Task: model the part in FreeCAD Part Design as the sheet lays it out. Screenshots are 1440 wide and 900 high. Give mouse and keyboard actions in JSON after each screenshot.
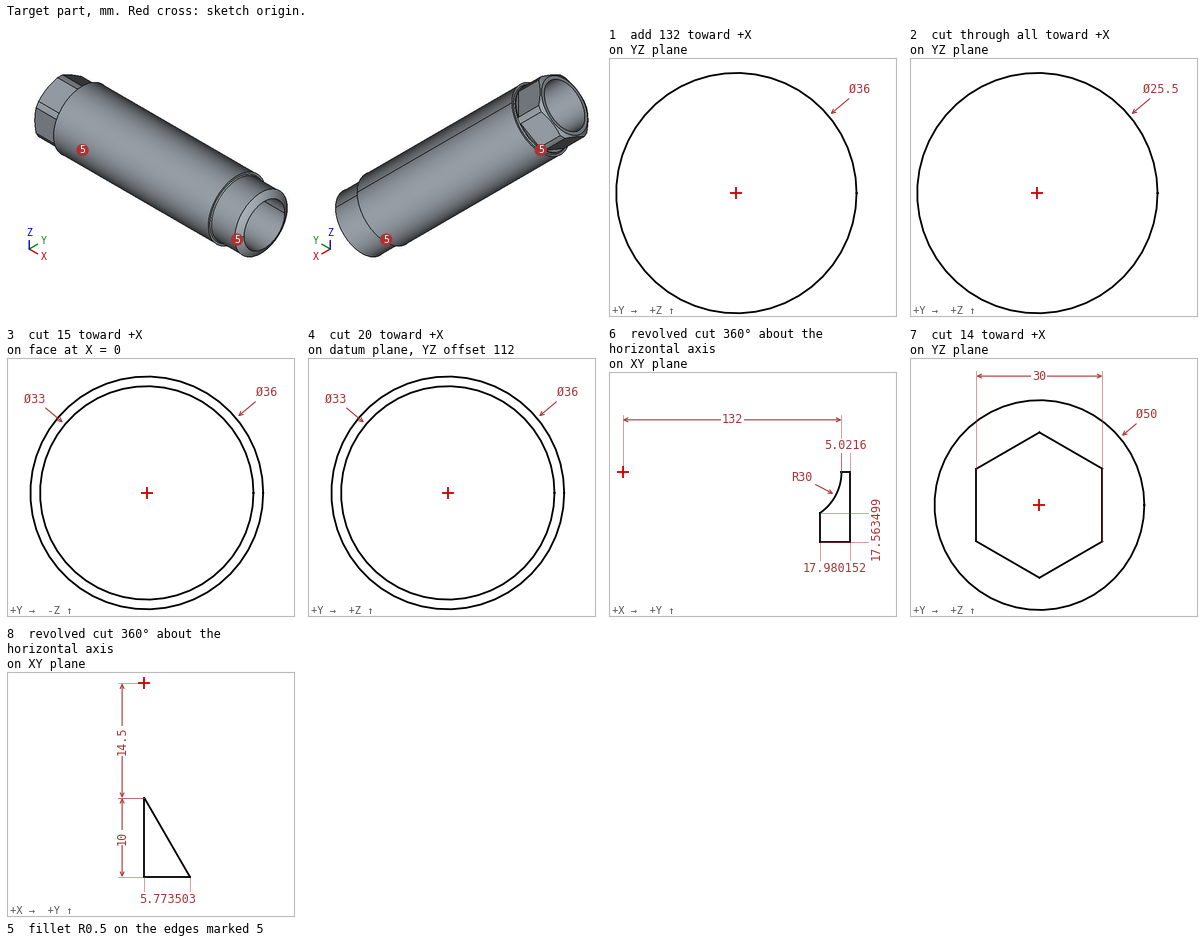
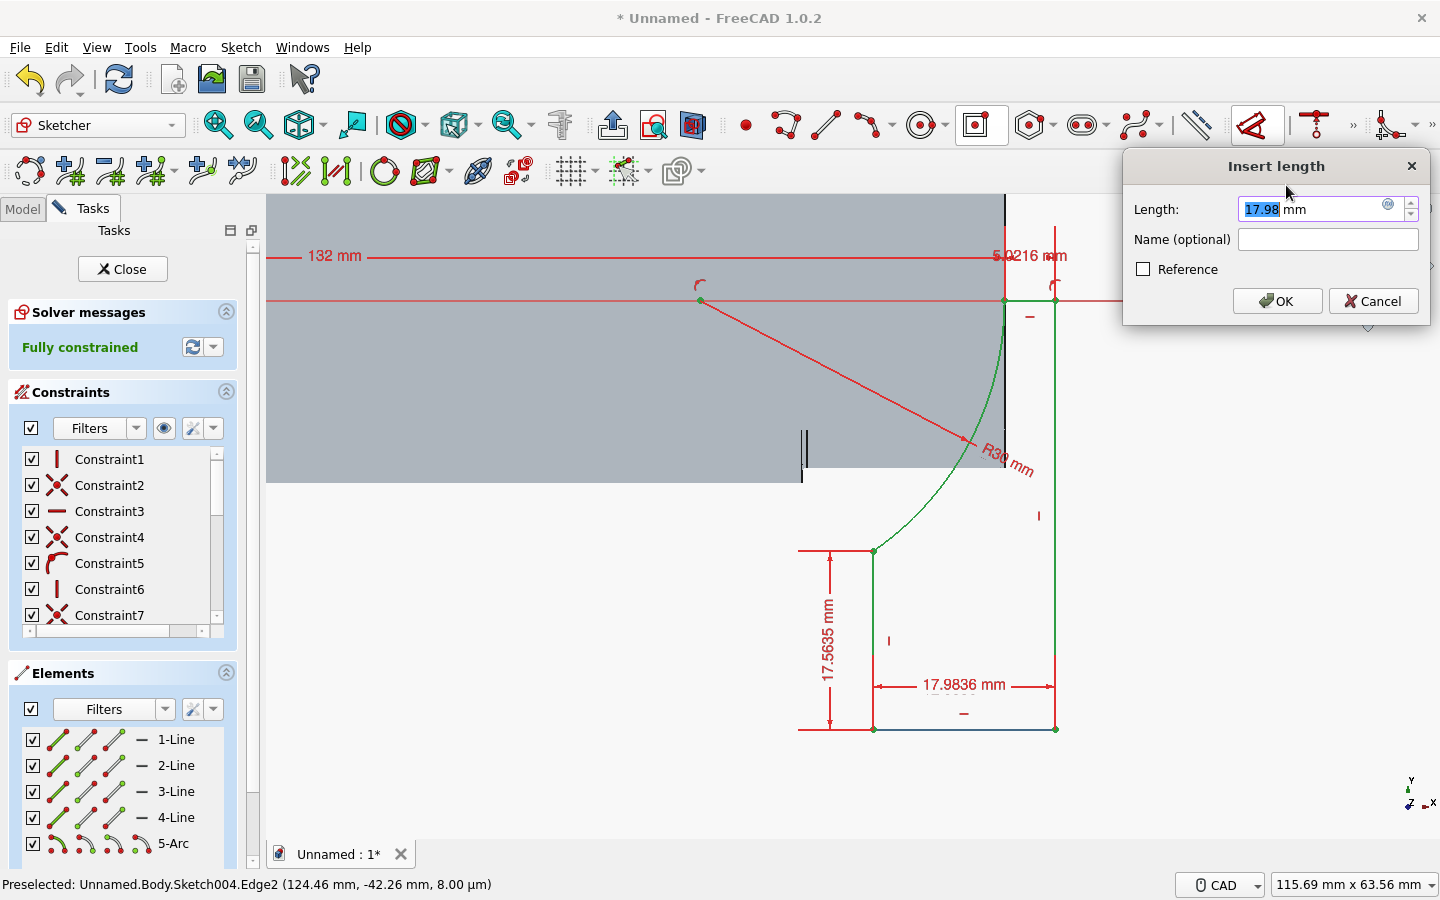
{"action": "type", "text": "17.980152"}
{"action": "key", "text": "Return"}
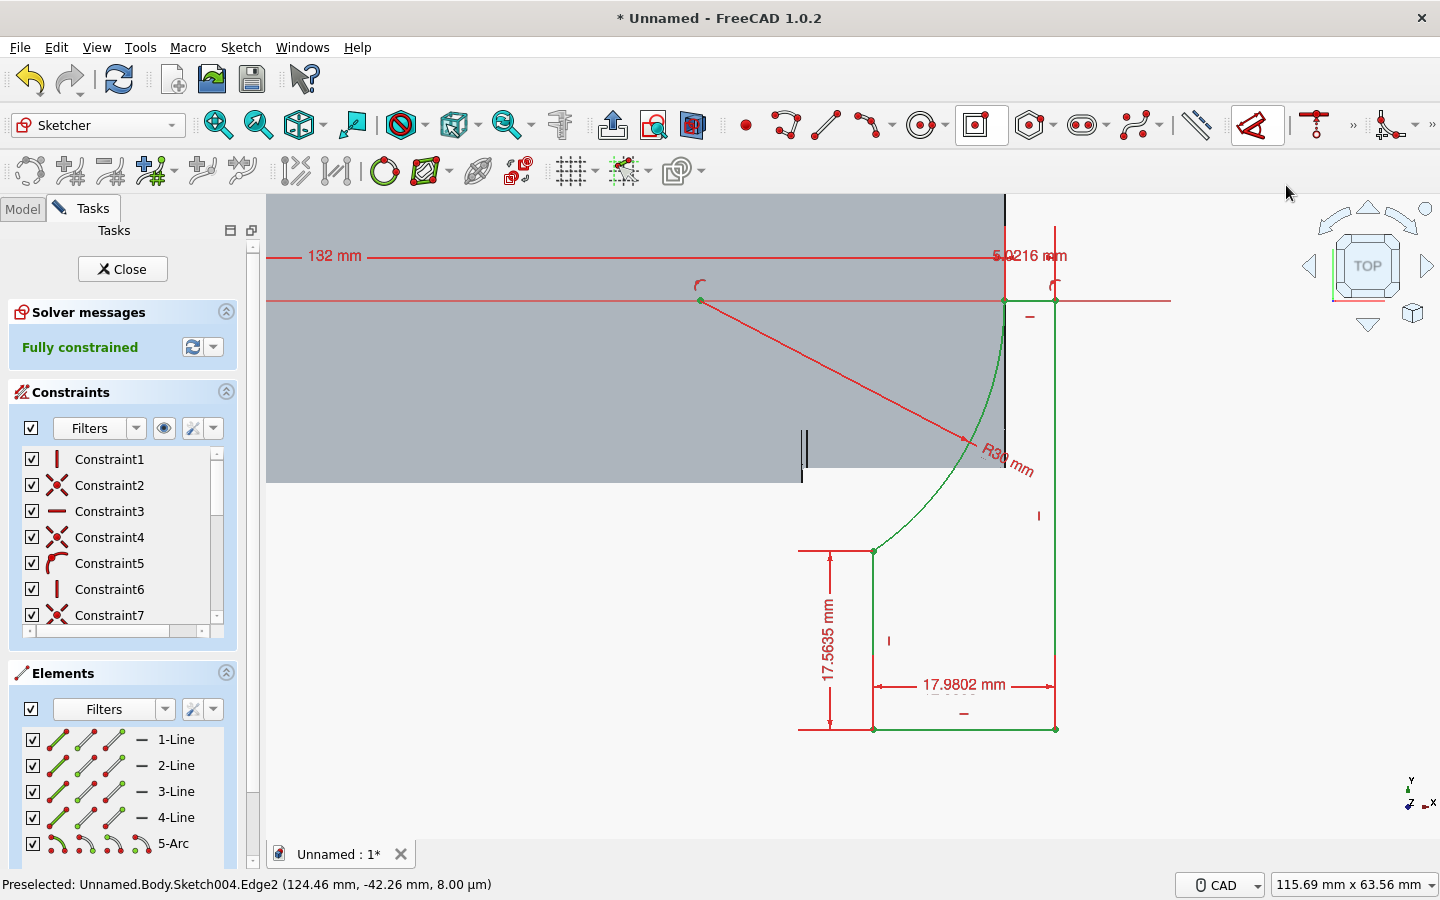
{"action": "left_click", "coordinate": [123, 269]}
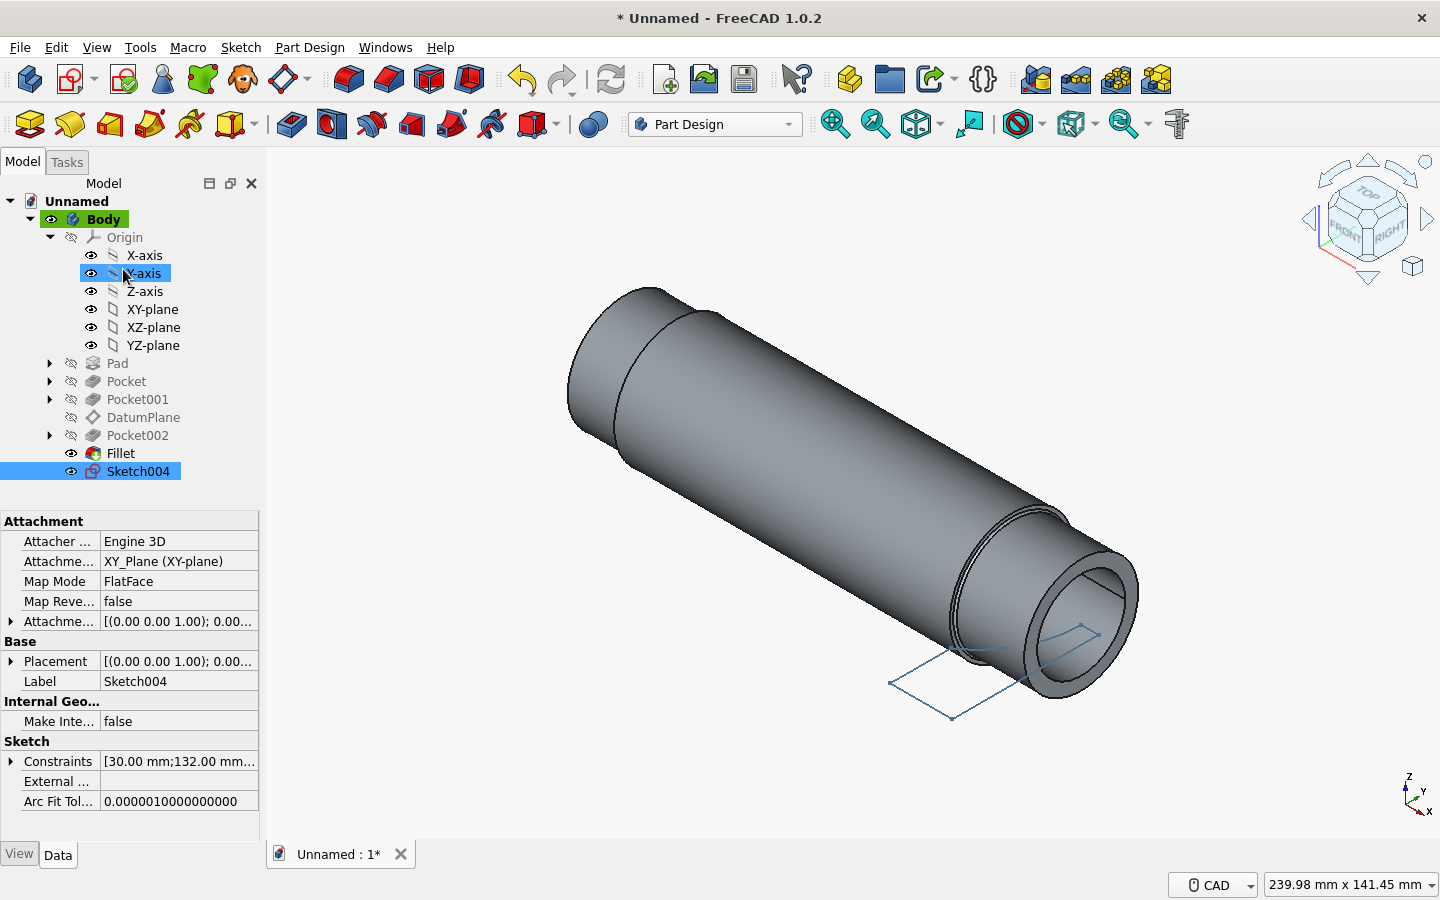
{"action": "left_click", "coordinate": [372, 124]}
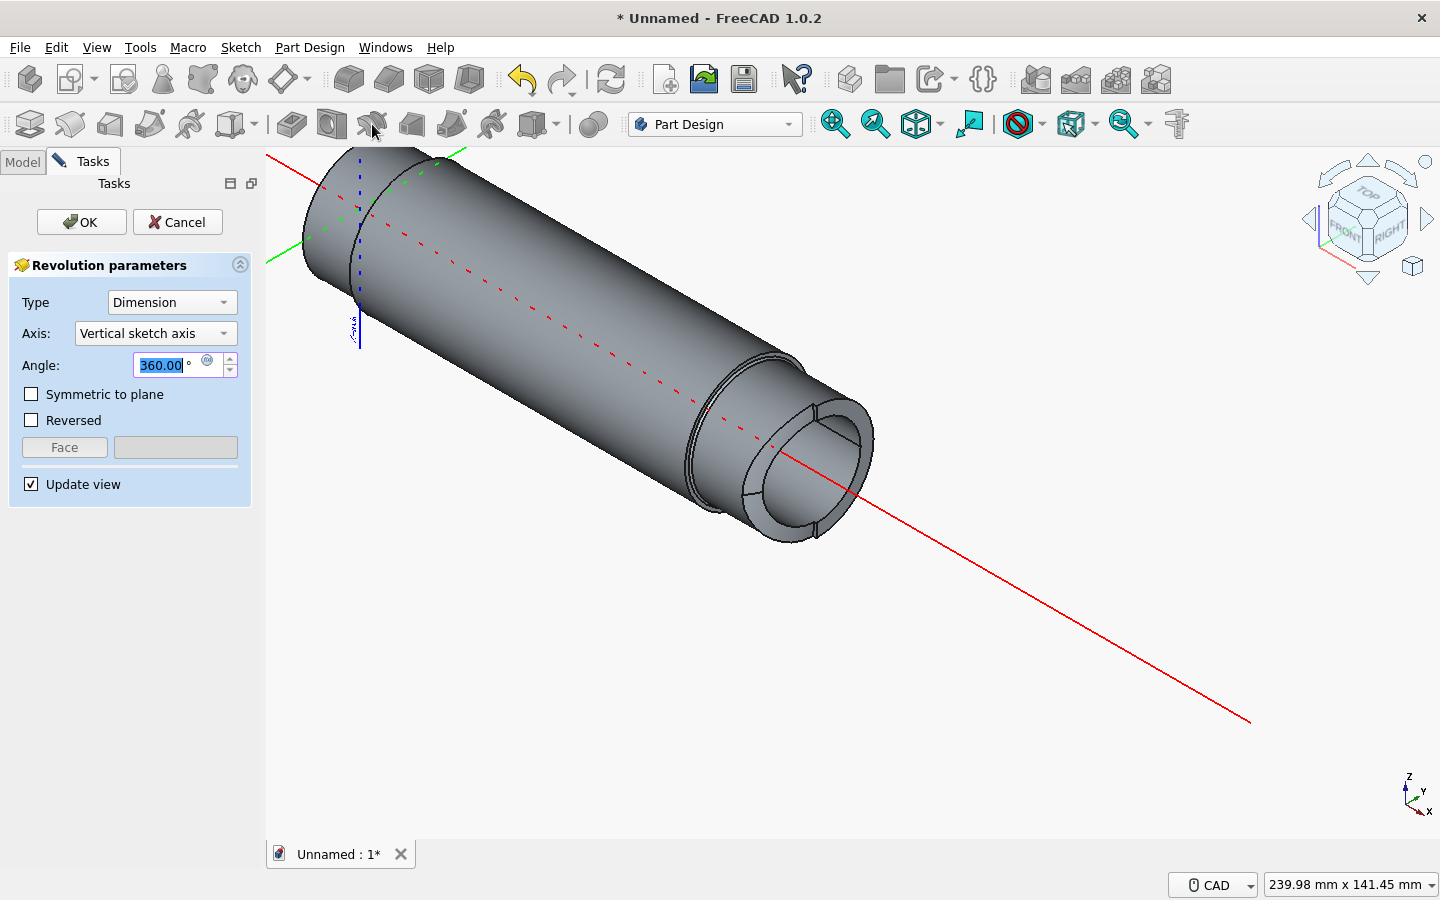
{"action": "left_click", "coordinate": [156, 334]}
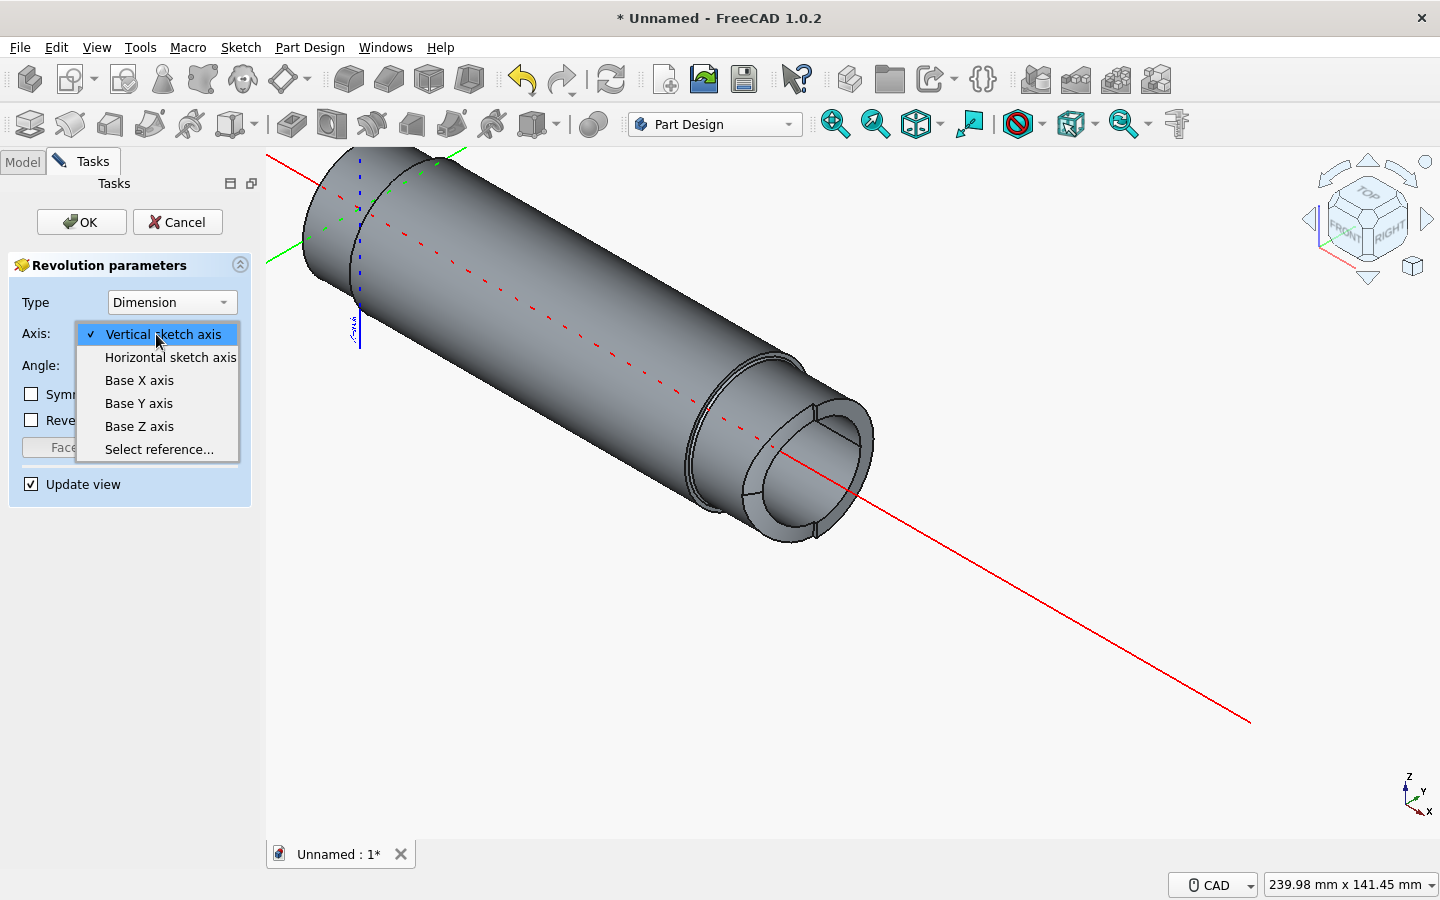
{"action": "left_click", "coordinate": [156, 358]}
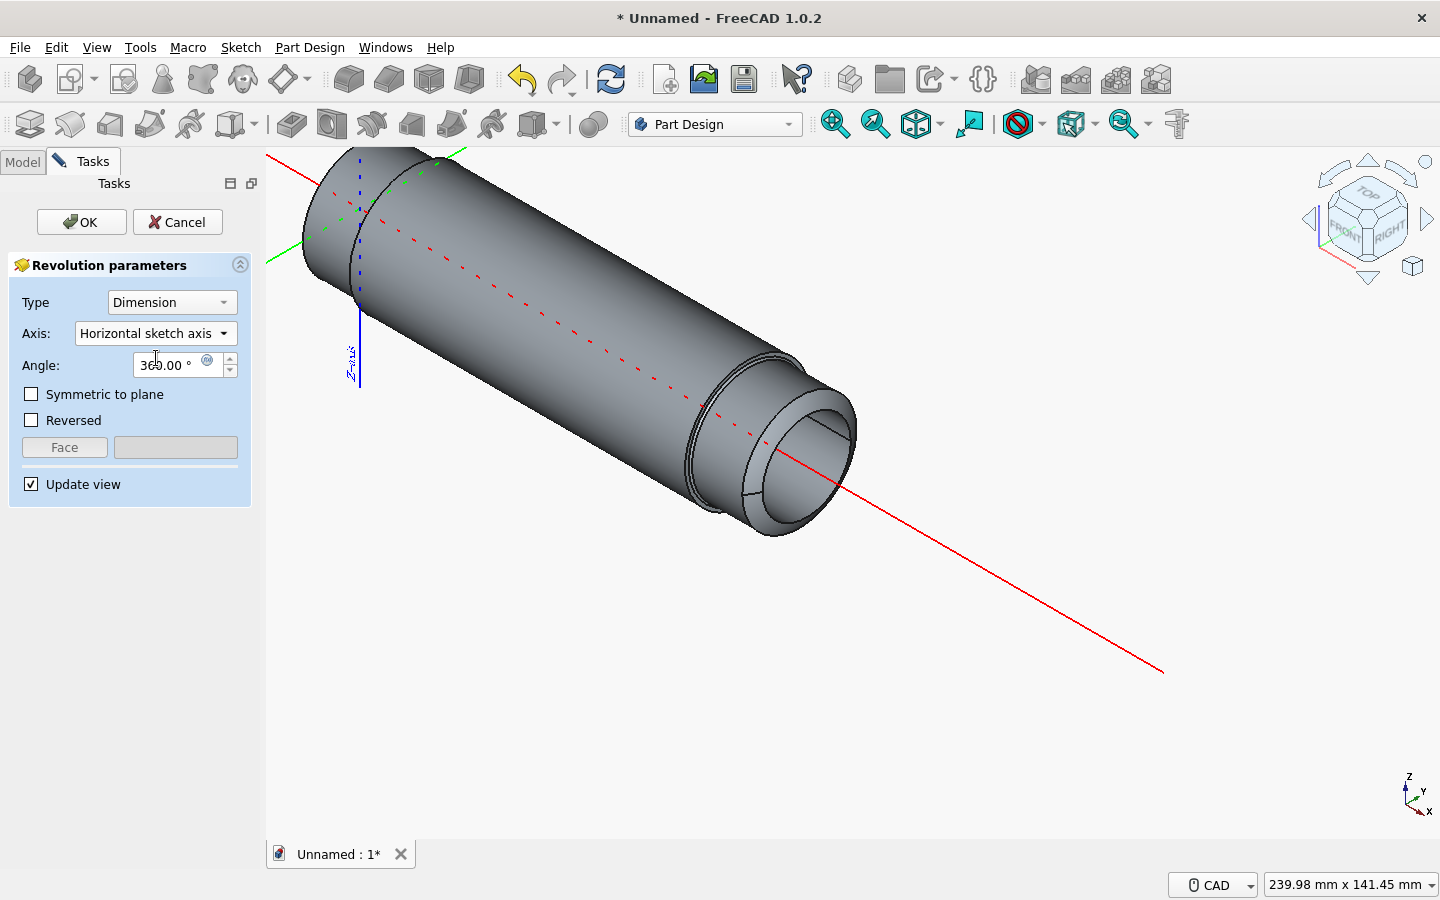
{"action": "left_click", "coordinate": [82, 222]}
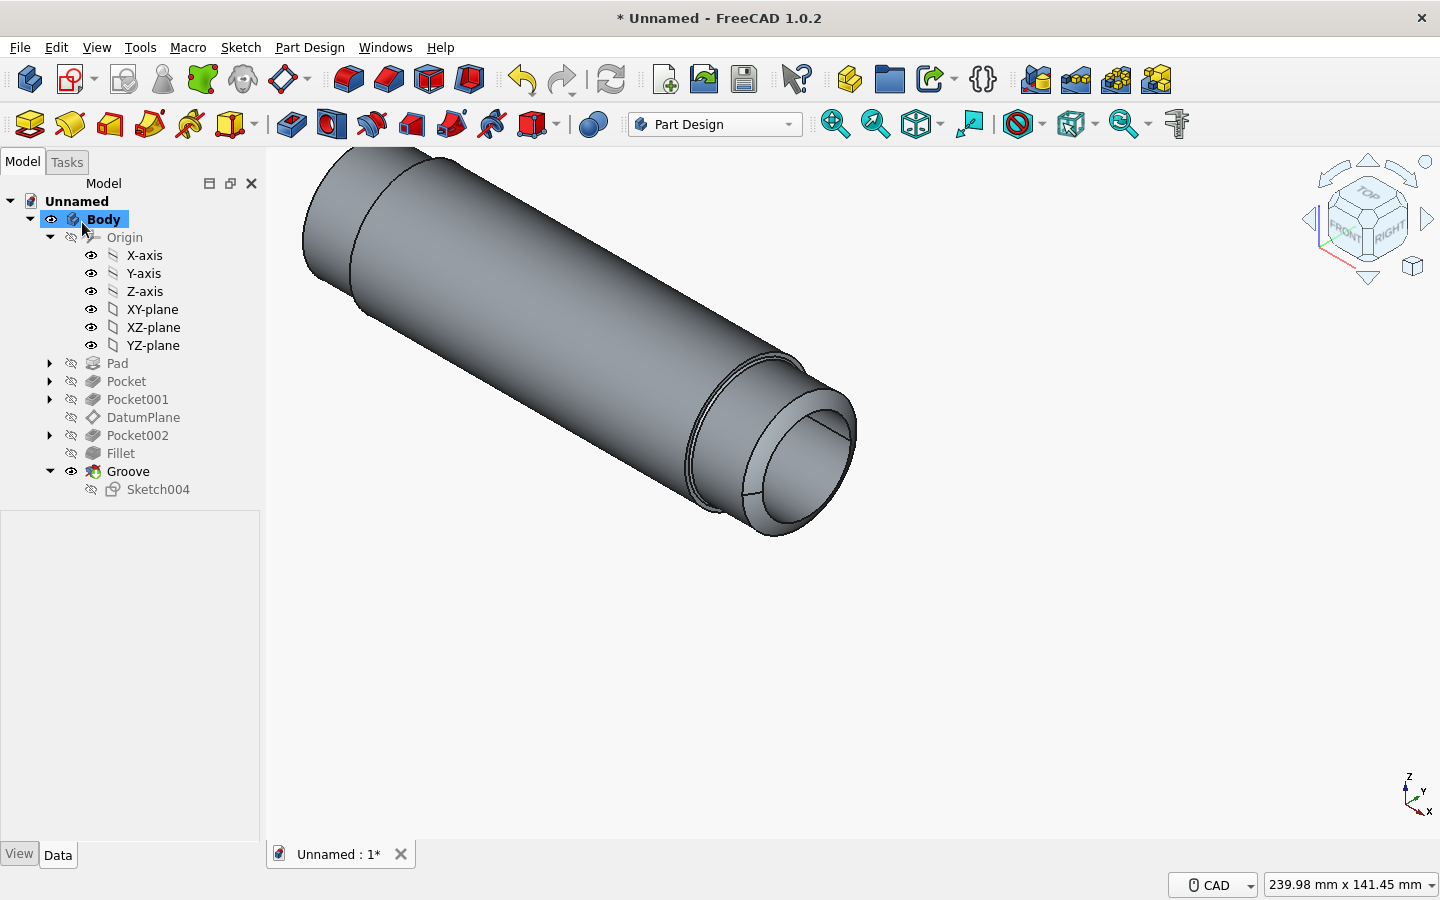
{"action": "left_click", "coordinate": [836, 124]}